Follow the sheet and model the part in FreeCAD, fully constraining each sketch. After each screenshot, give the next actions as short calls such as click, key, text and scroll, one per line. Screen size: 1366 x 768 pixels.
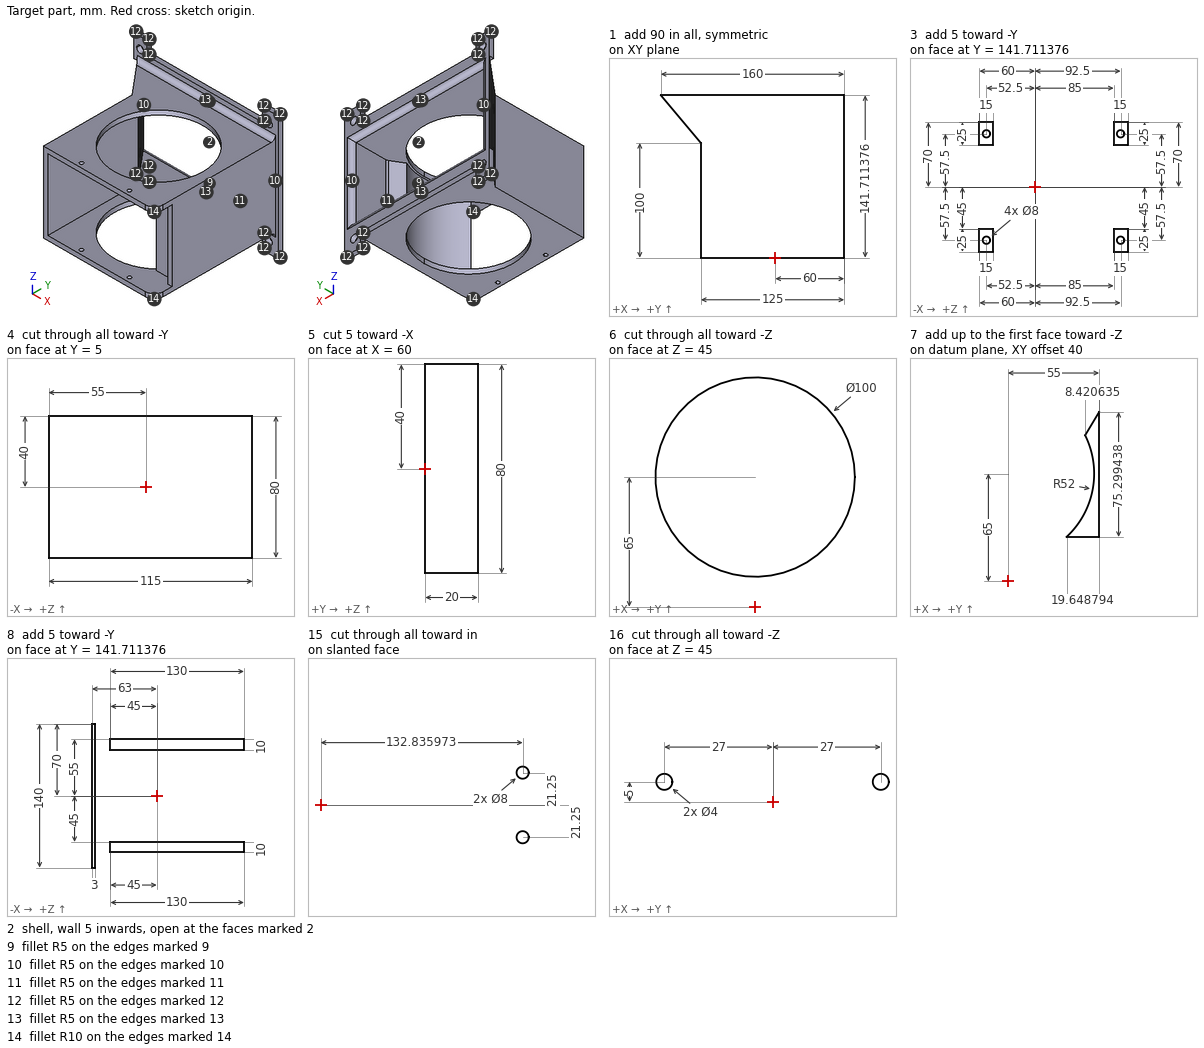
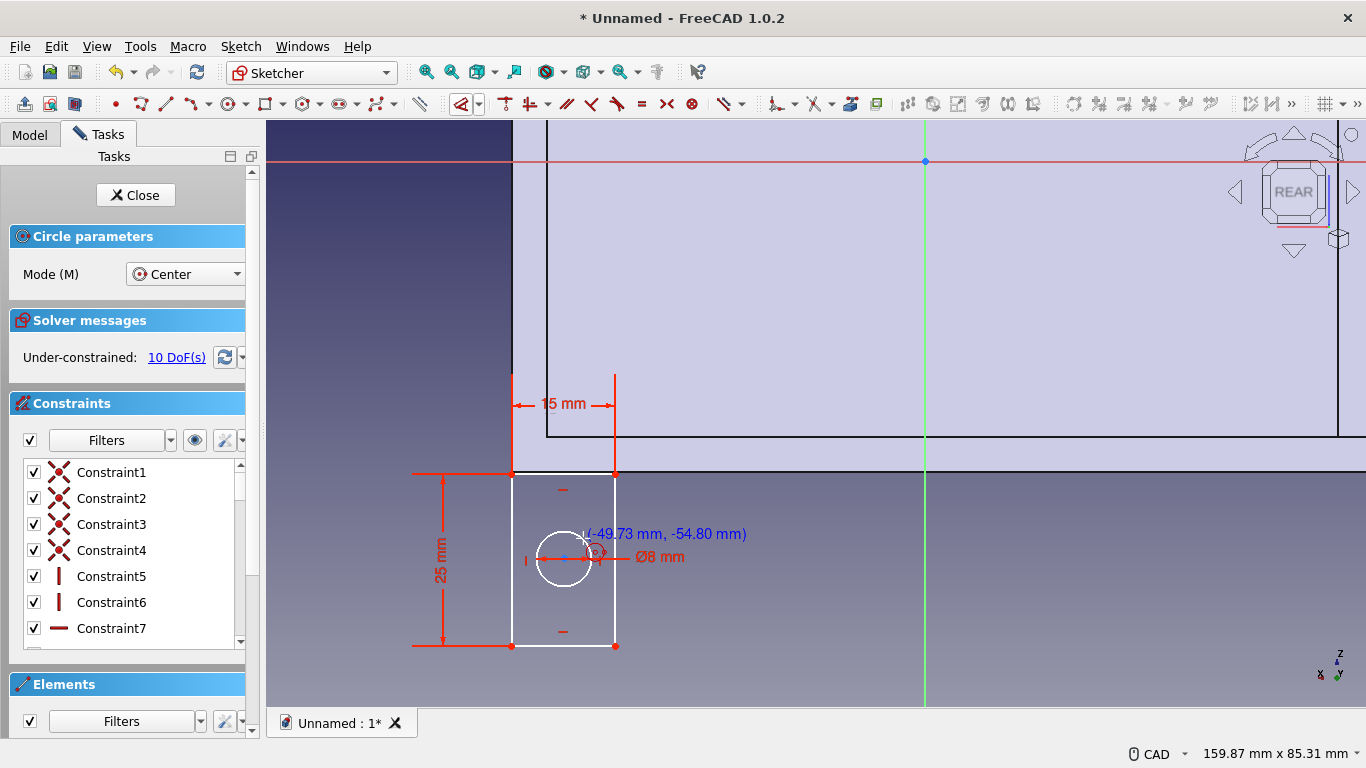
scroll(564, 560, down, 5)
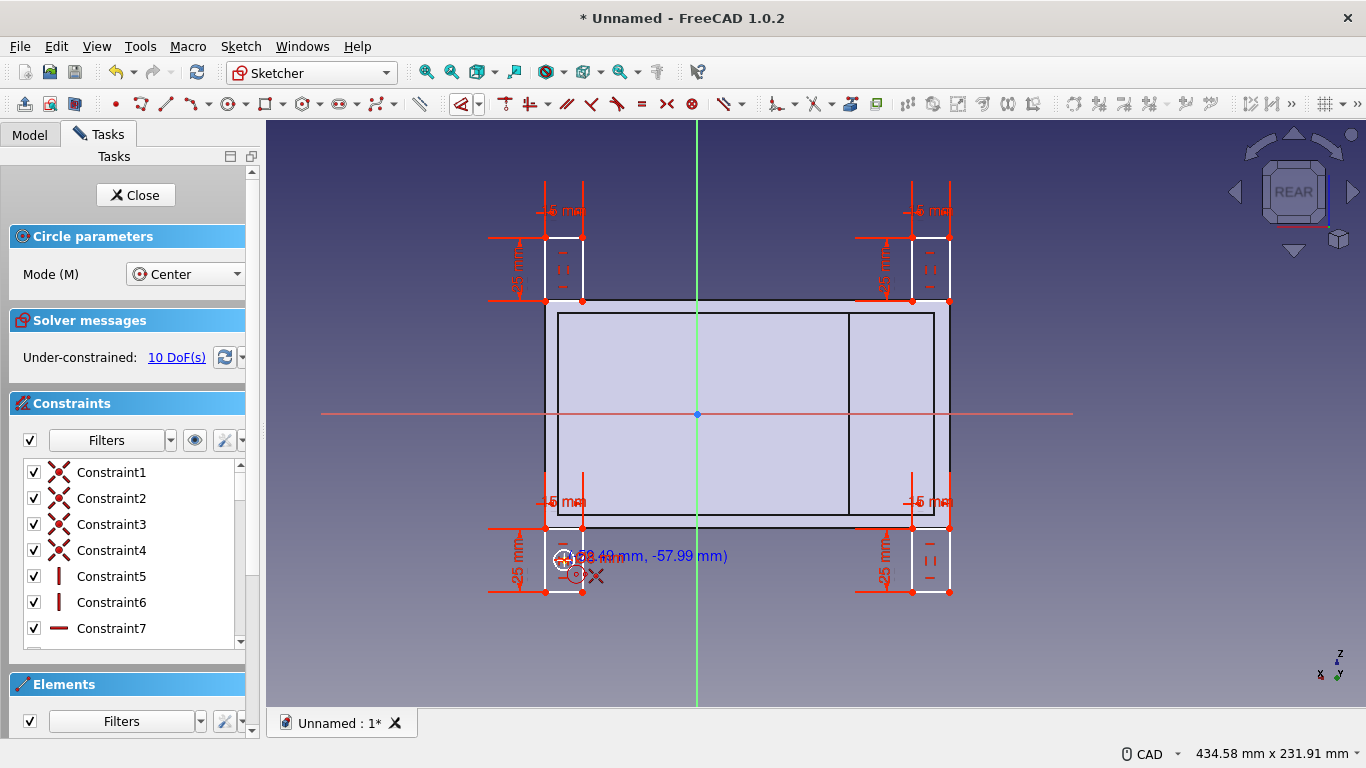
scroll(931, 269, up, 5)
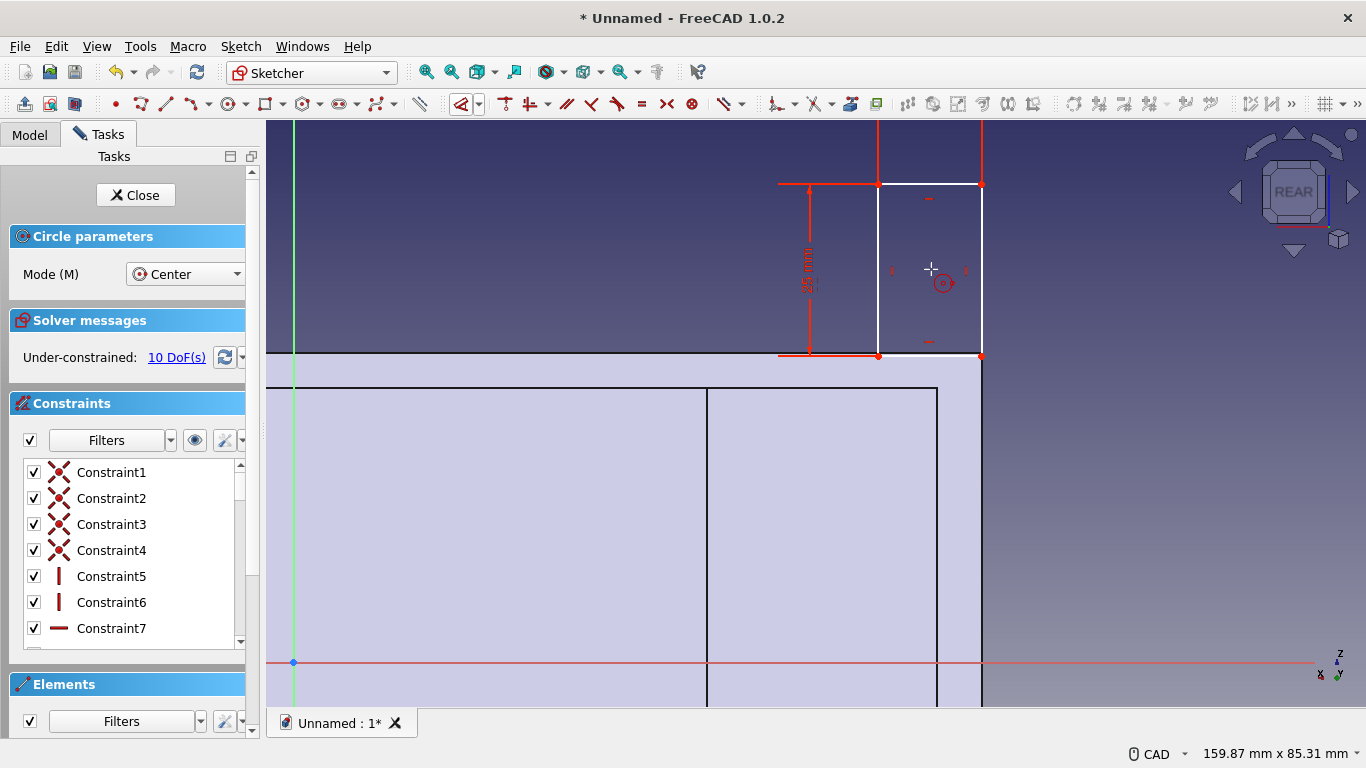
click(930, 267)
move(950, 248)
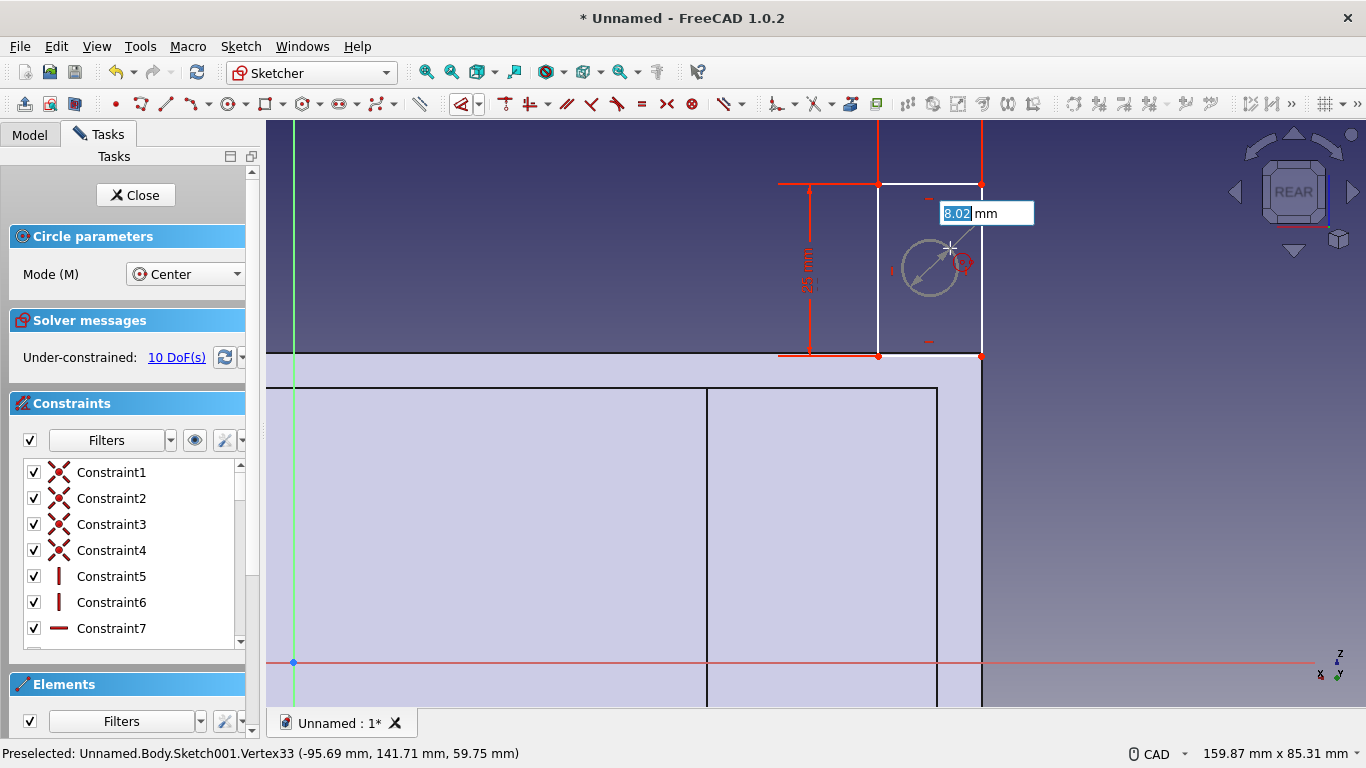
text(8)
key(Return)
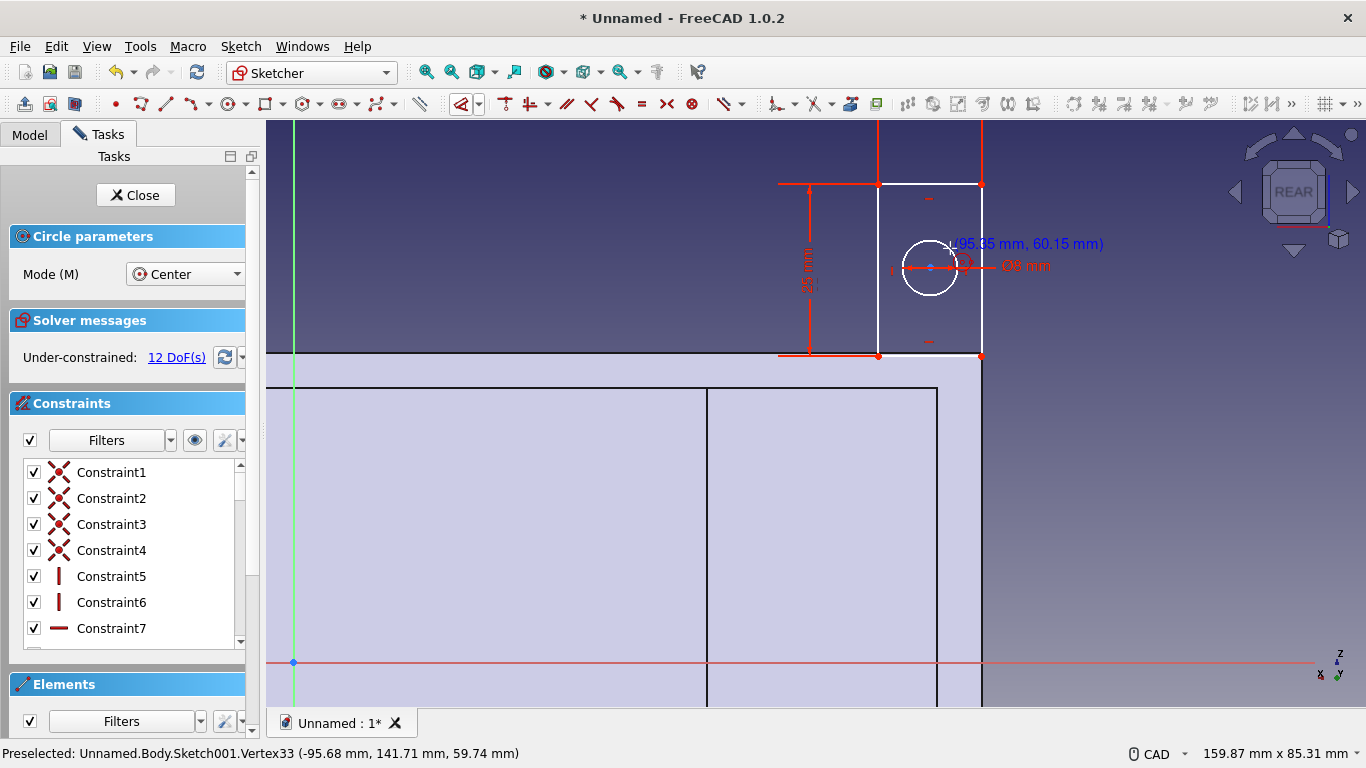
scroll(931, 268, down, 5)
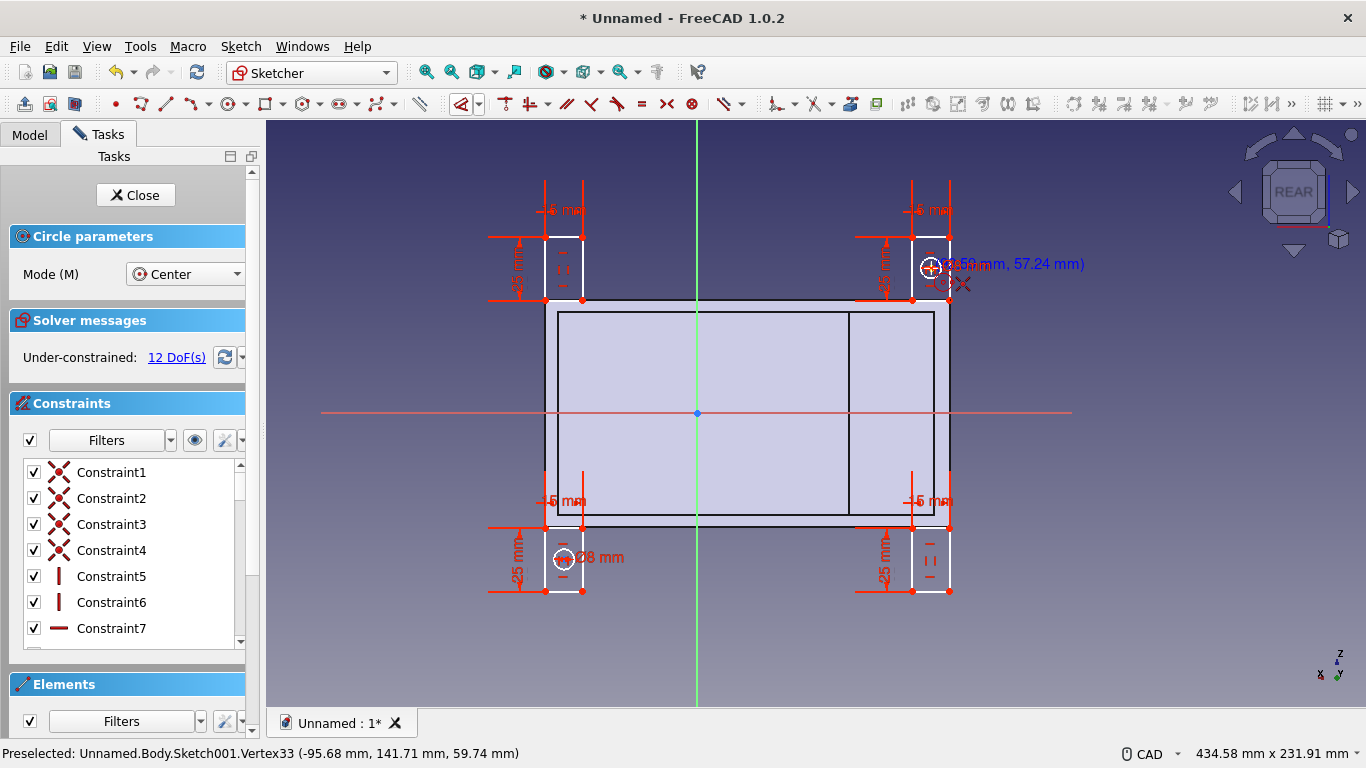
scroll(564, 268, up, 5)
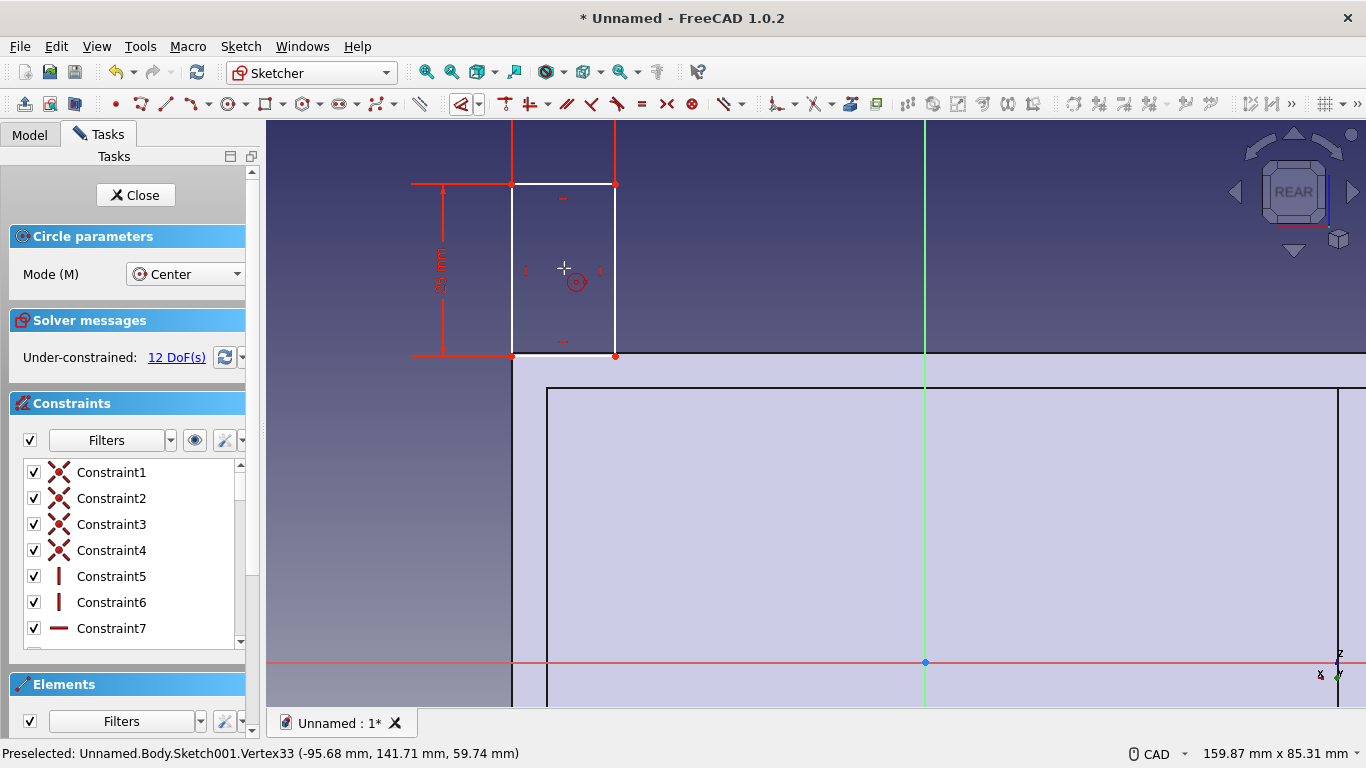
click(564, 267)
move(583, 248)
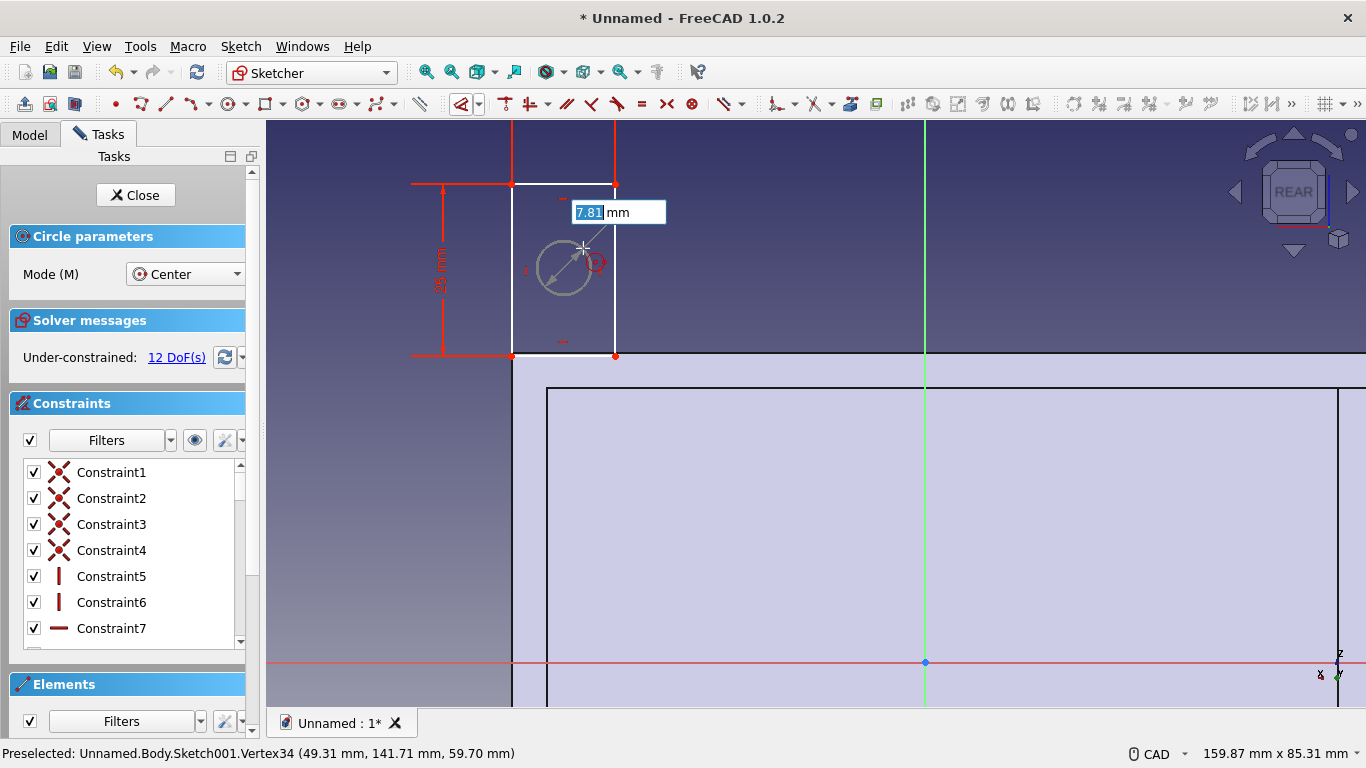
text(8)
key(Return)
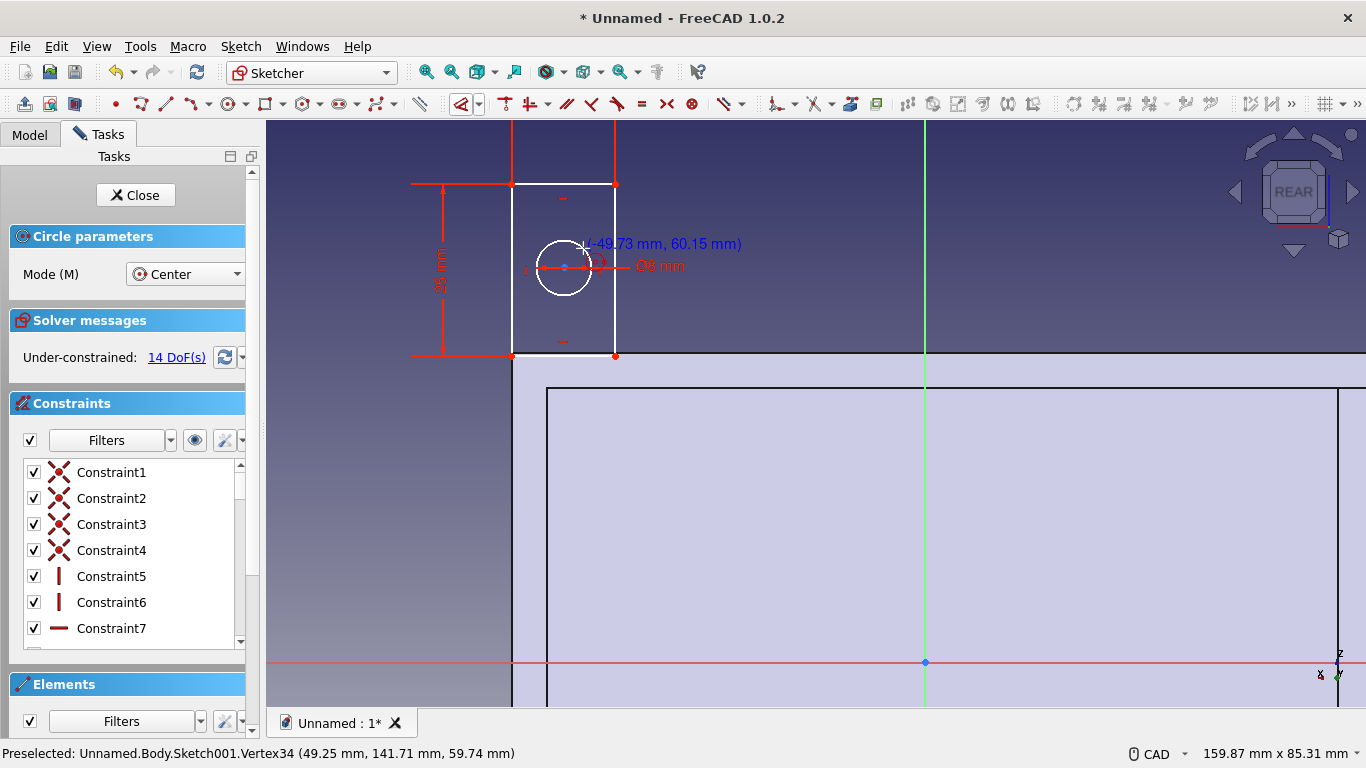
scroll(564, 268, down, 5)